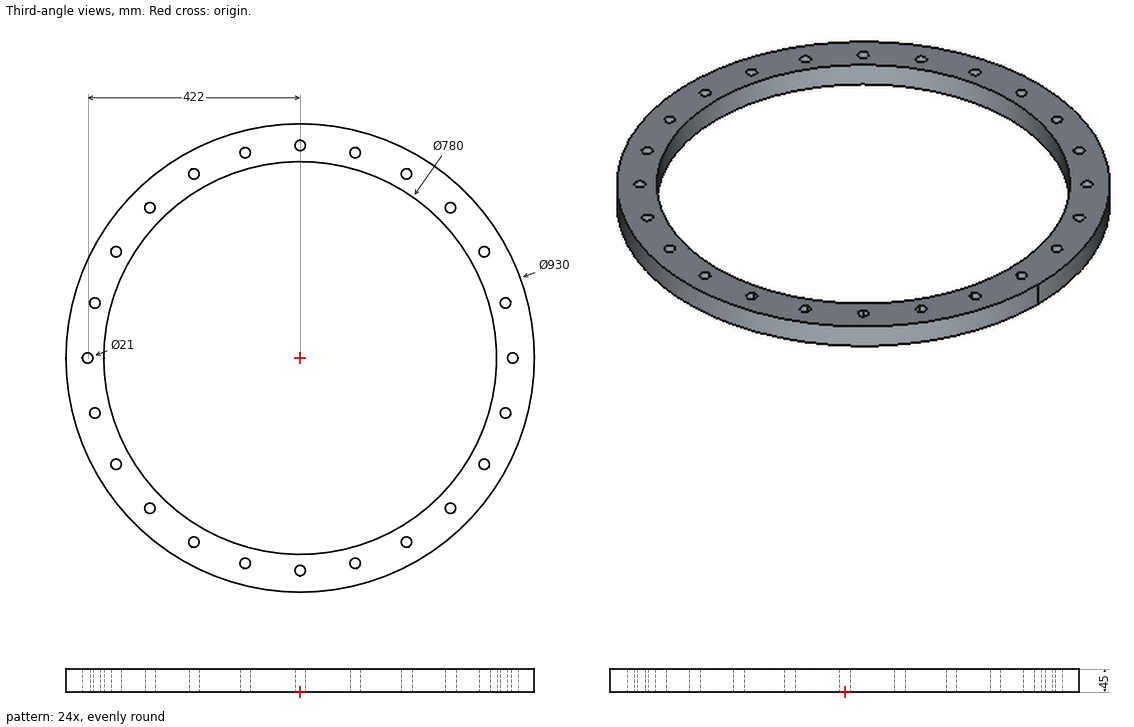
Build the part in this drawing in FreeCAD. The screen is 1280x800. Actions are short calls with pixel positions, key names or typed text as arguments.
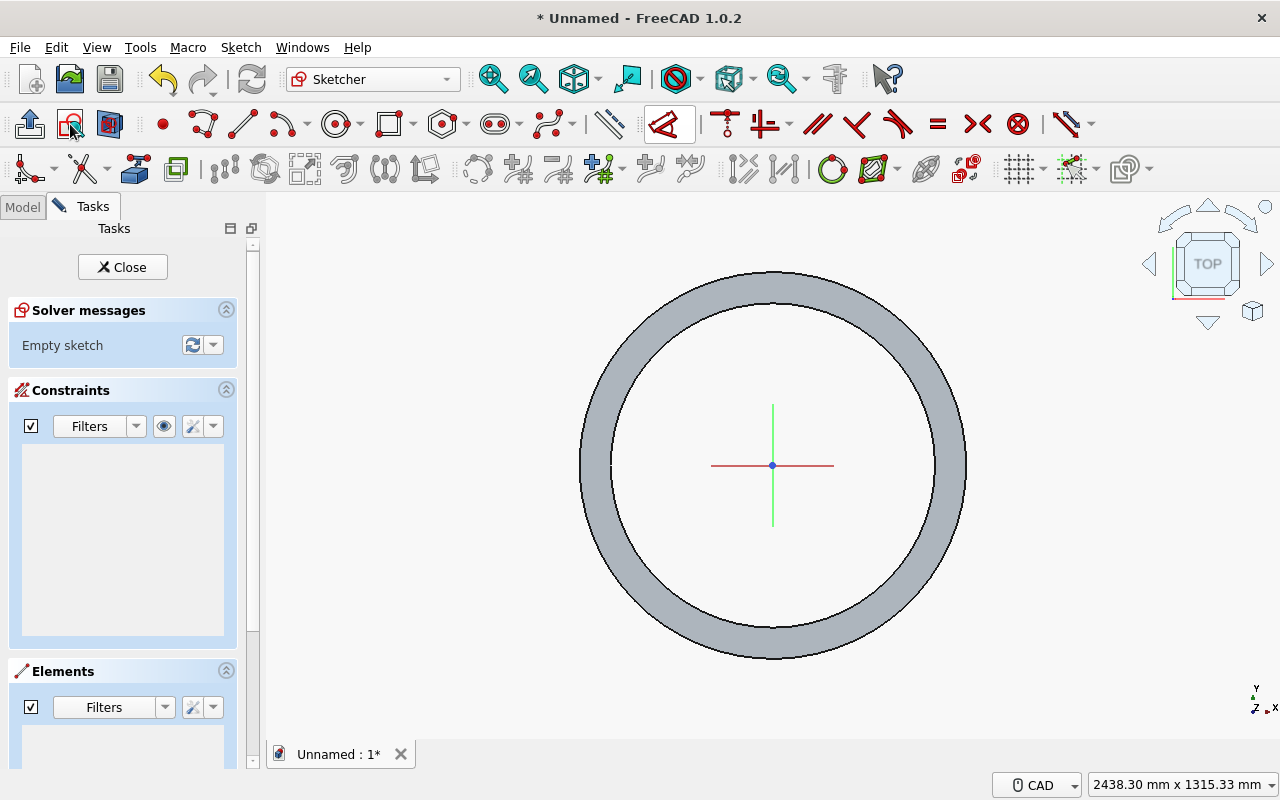
scroll(592, 466, up, 15)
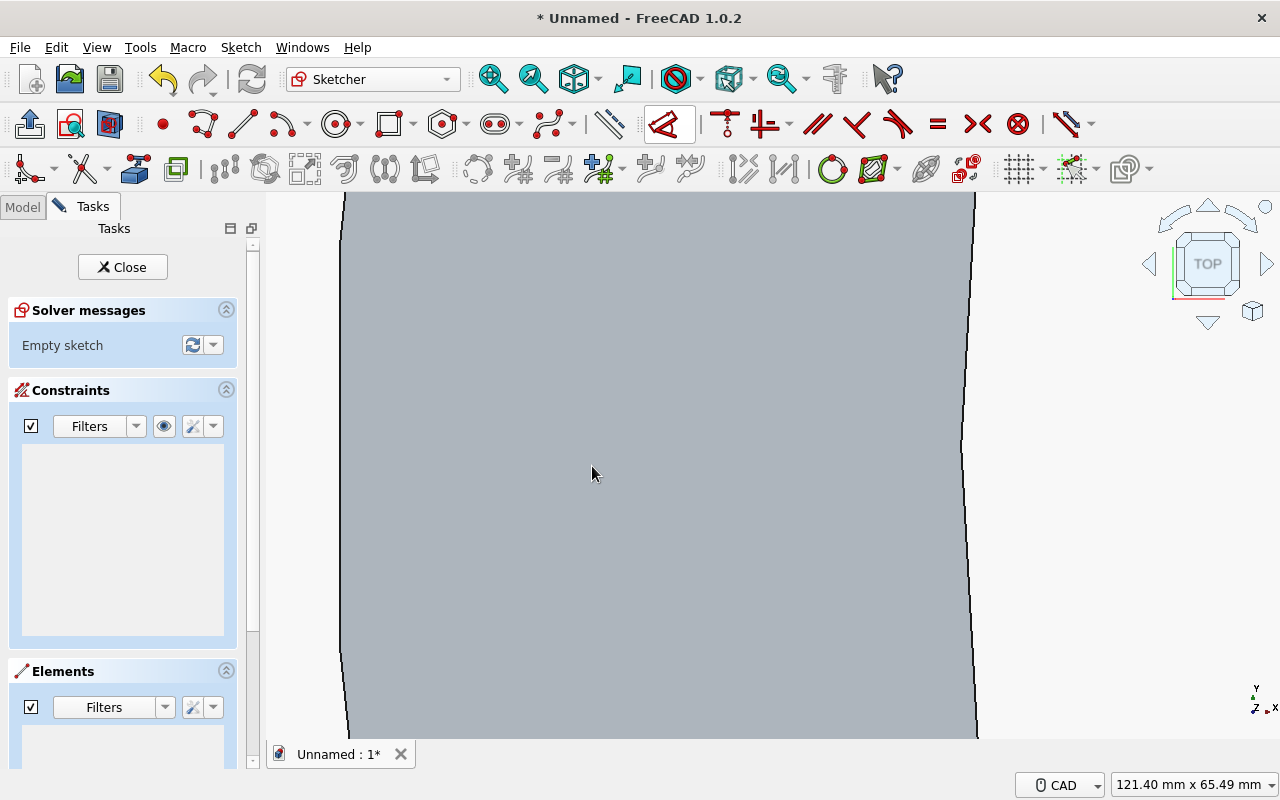
scroll(681, 423, up, 3)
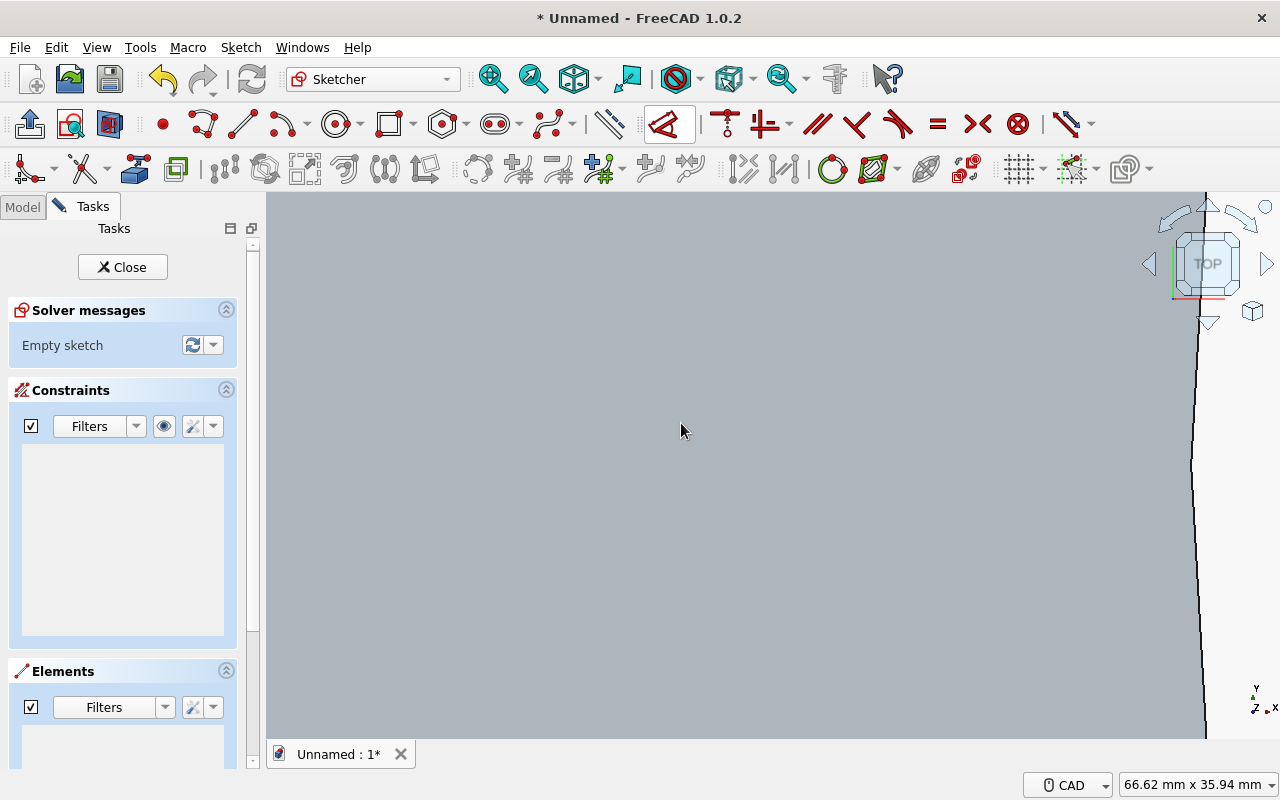
click(336, 124)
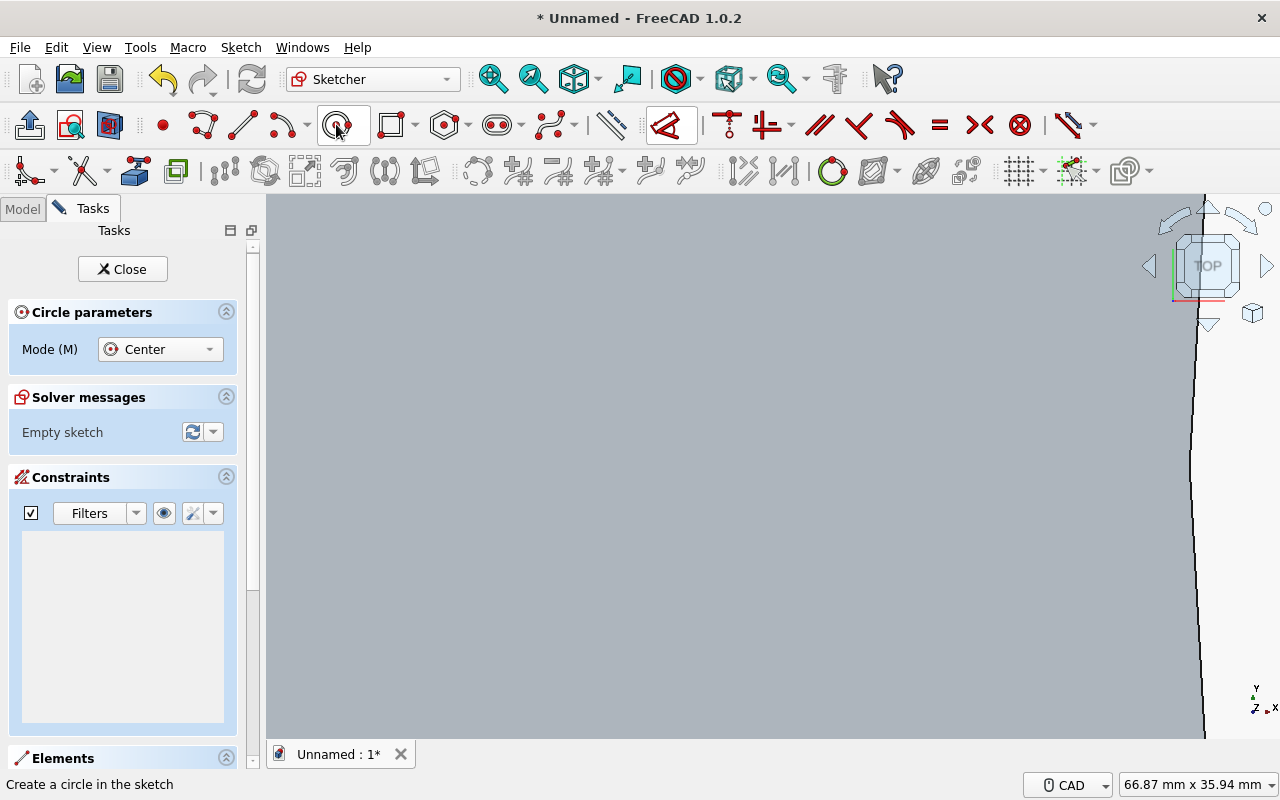
click(704, 466)
click(817, 354)
key(Escape)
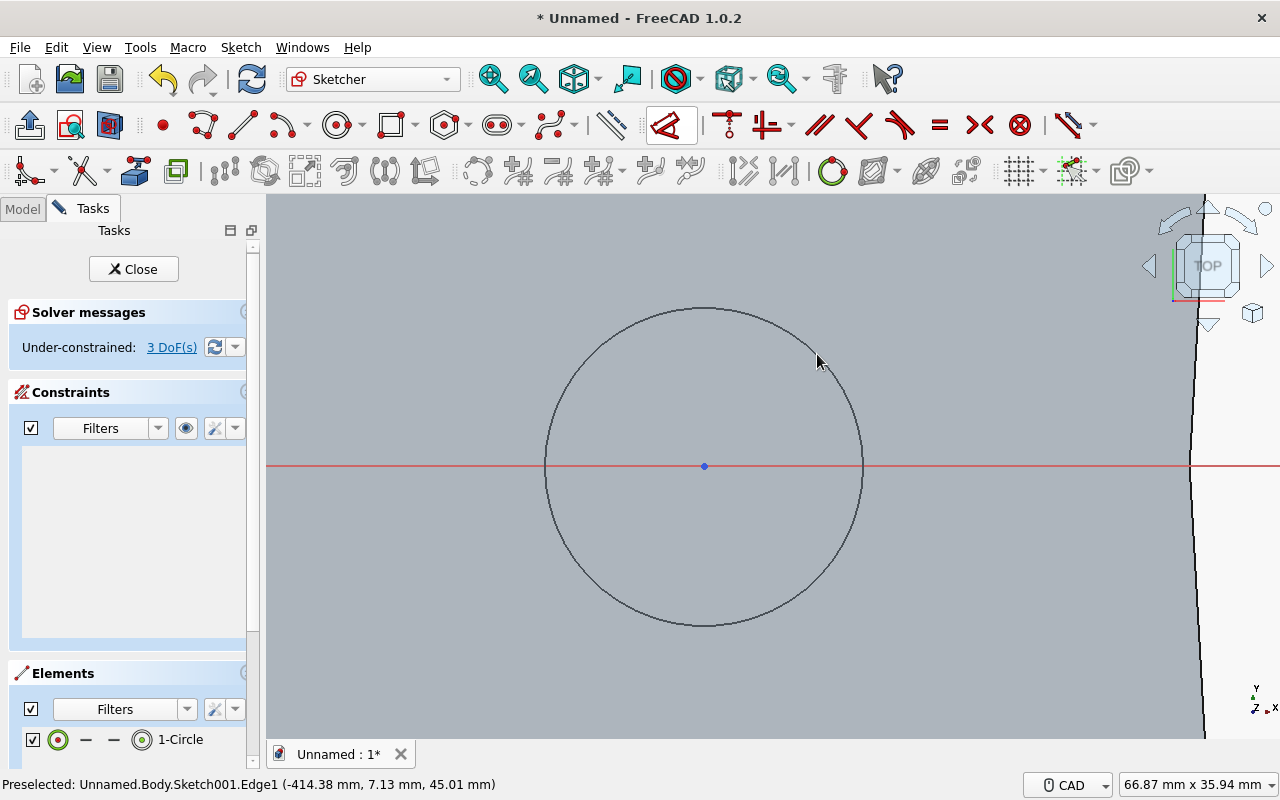
click(704, 467)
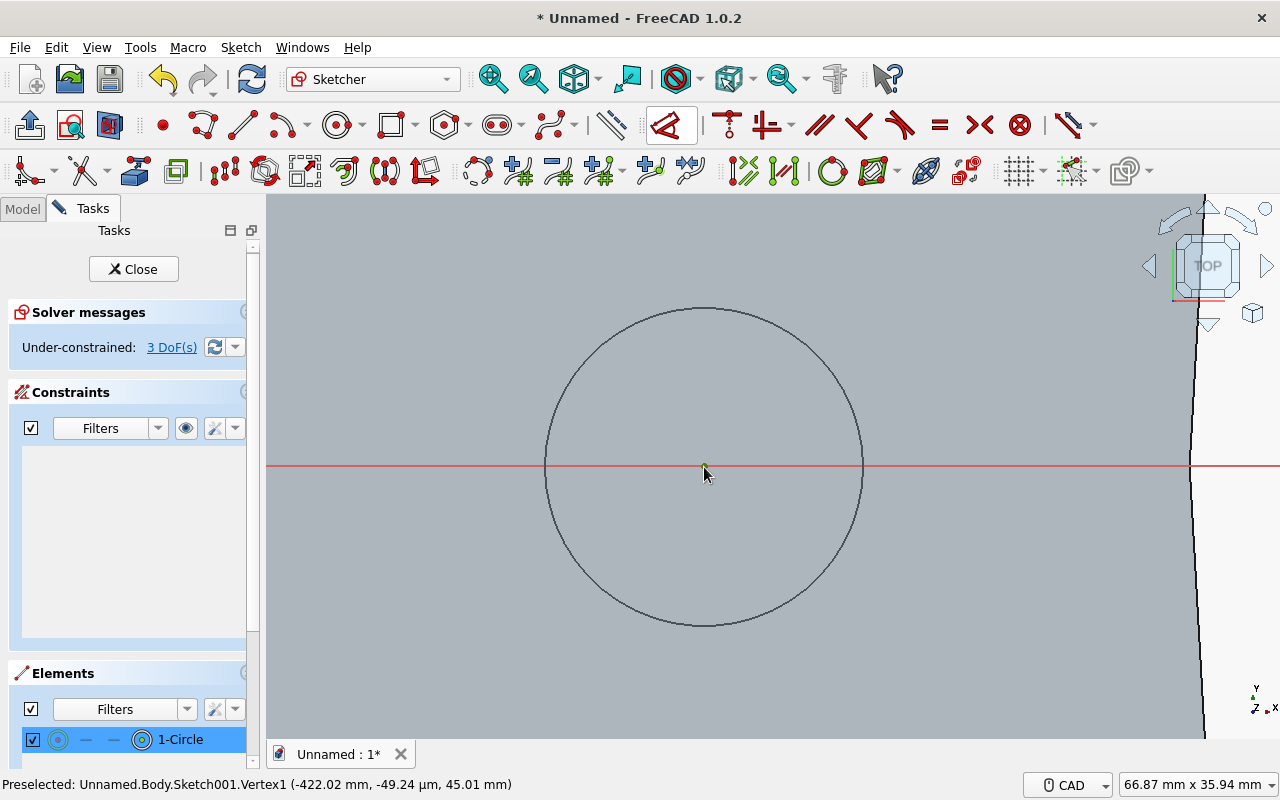
click(353, 466)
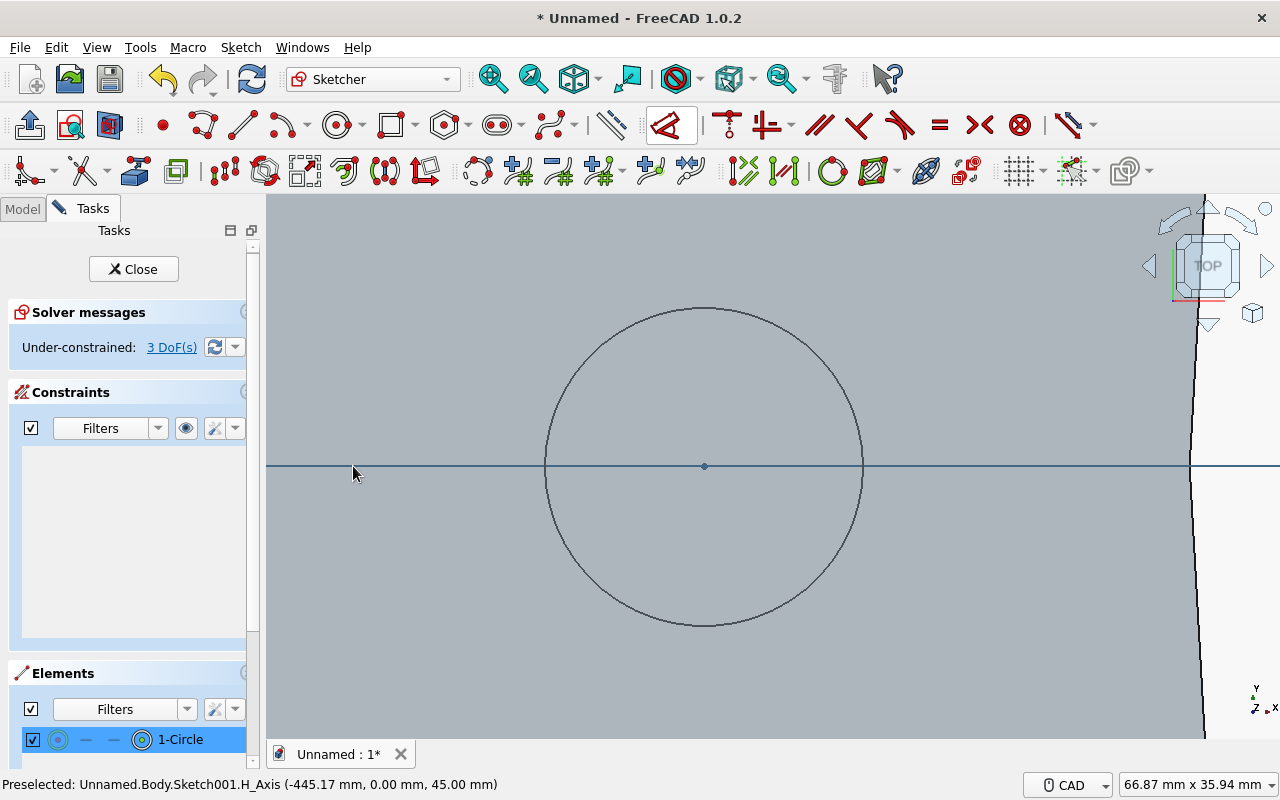
click(728, 126)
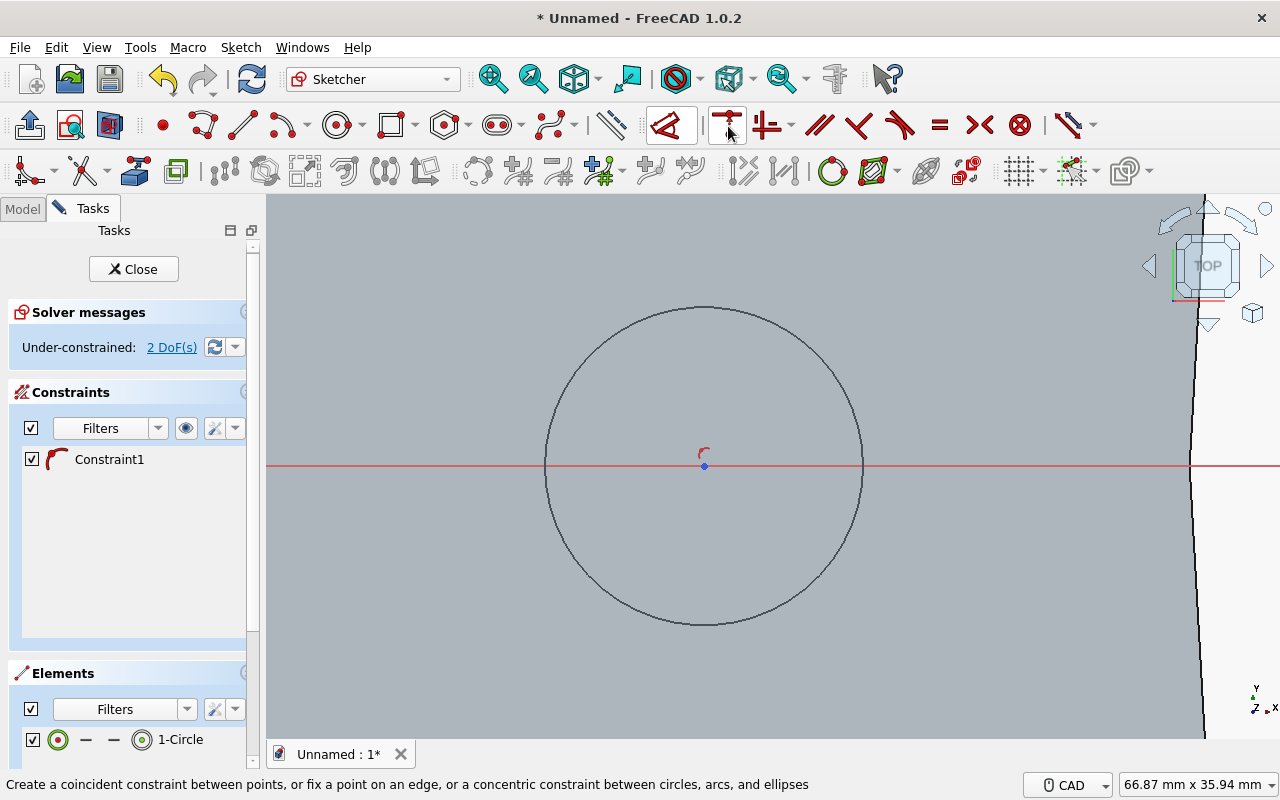
click(666, 126)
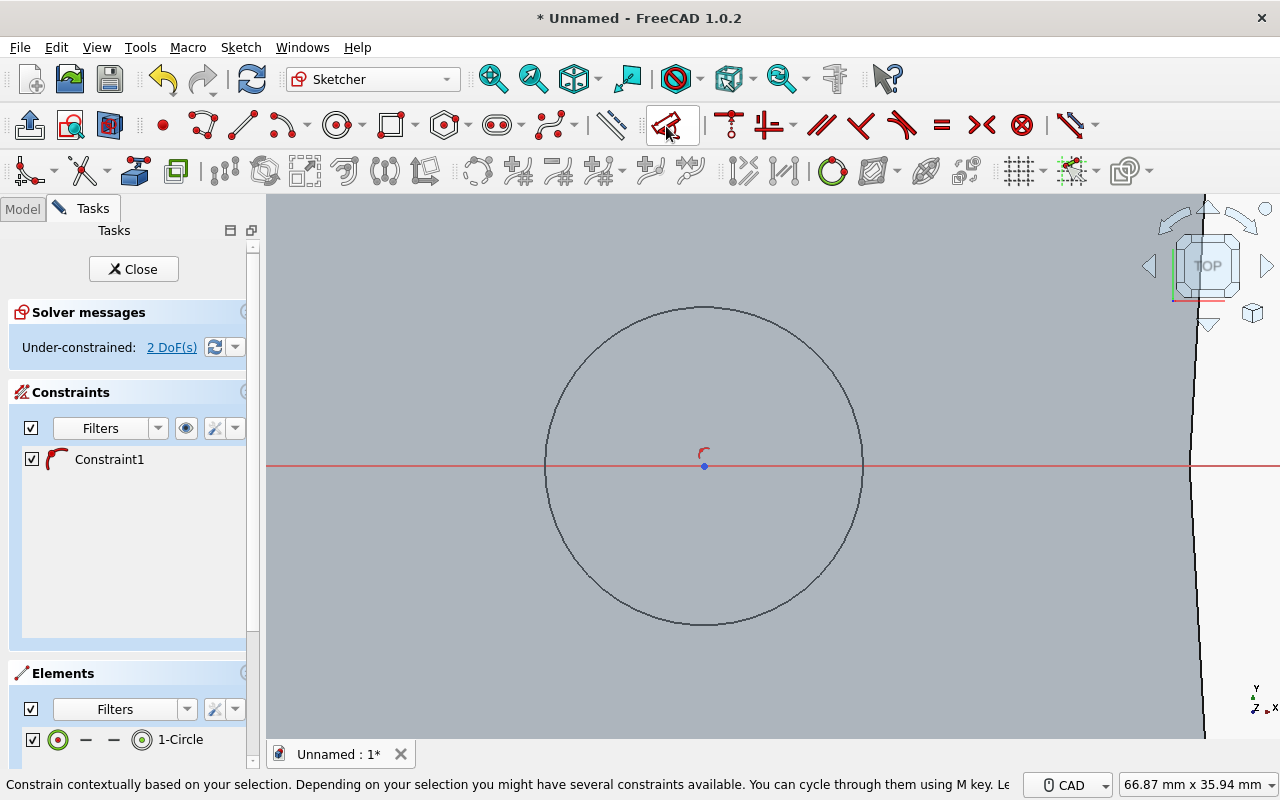
click(816, 353)
click(839, 330)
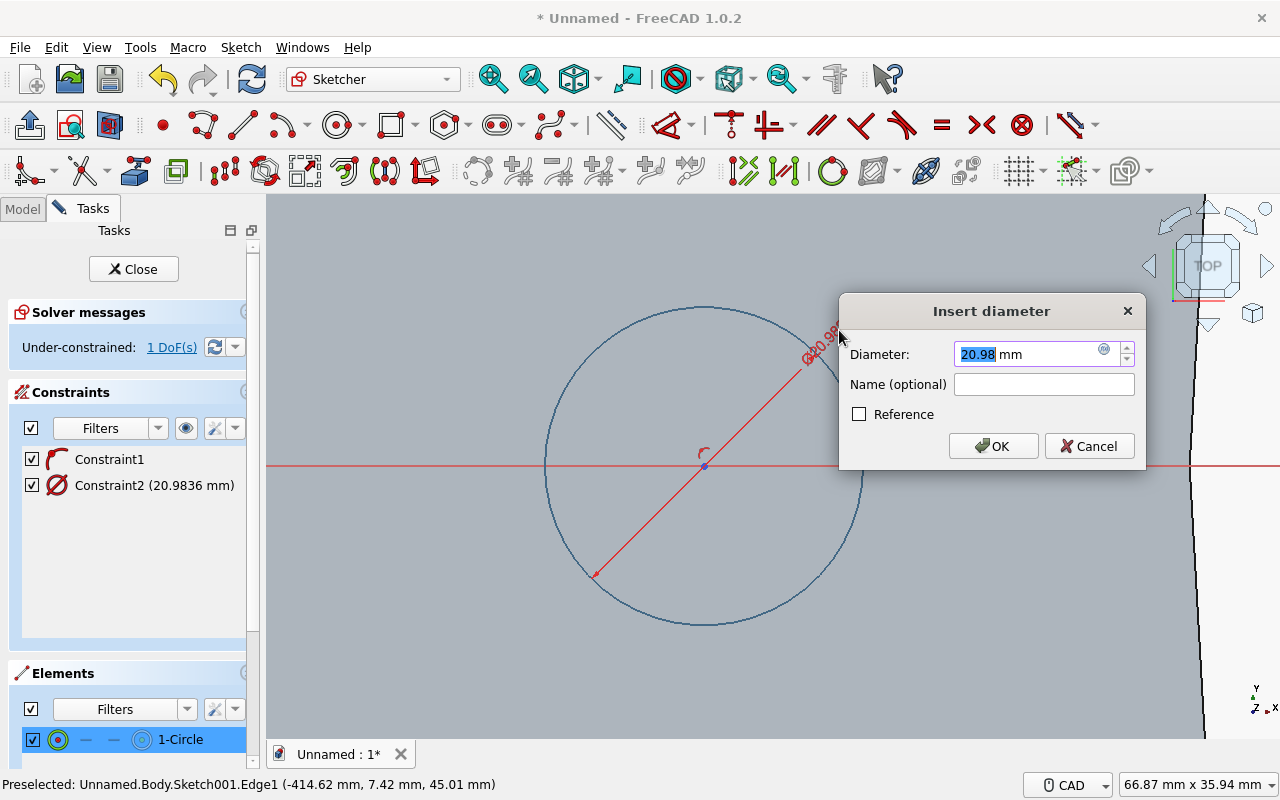
text(21)
key(Return)